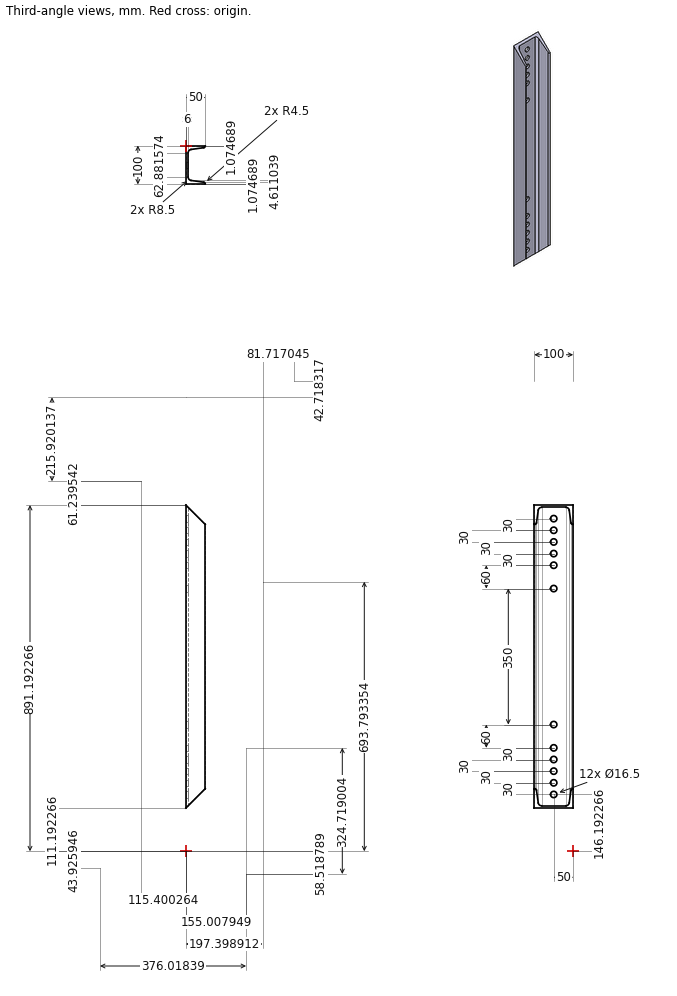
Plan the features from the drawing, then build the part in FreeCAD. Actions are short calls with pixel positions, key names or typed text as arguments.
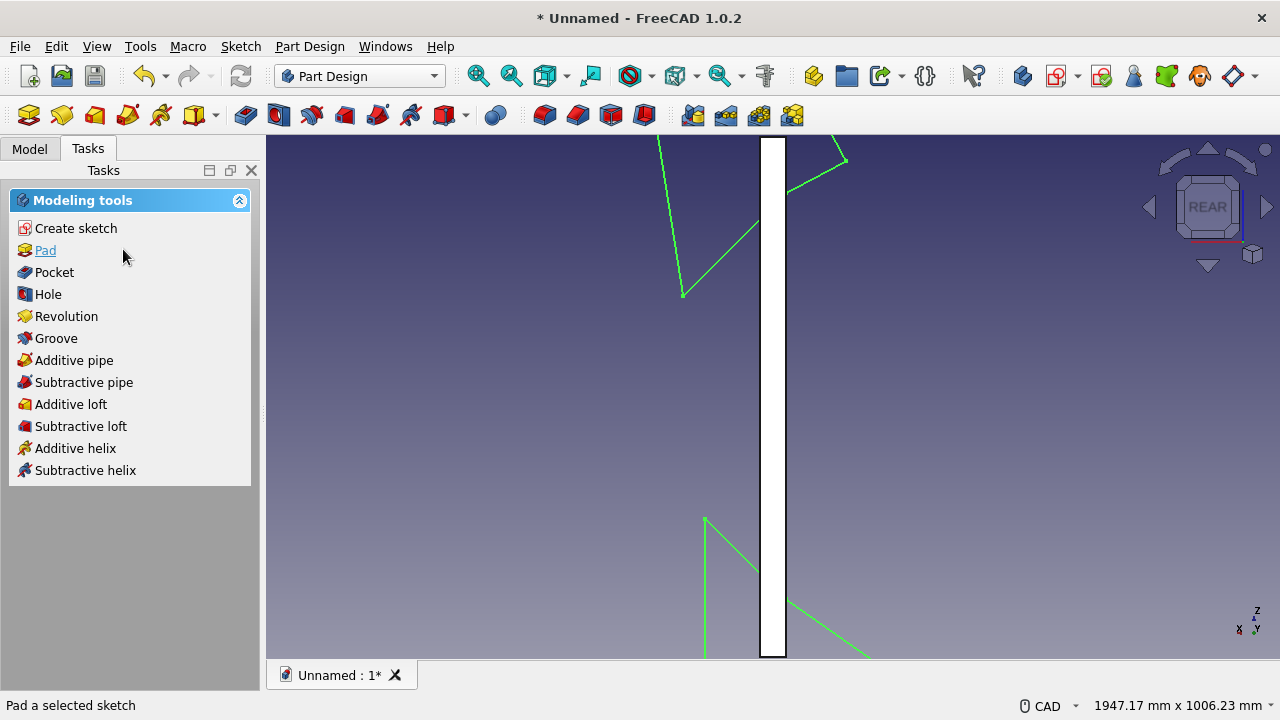
click(246, 116)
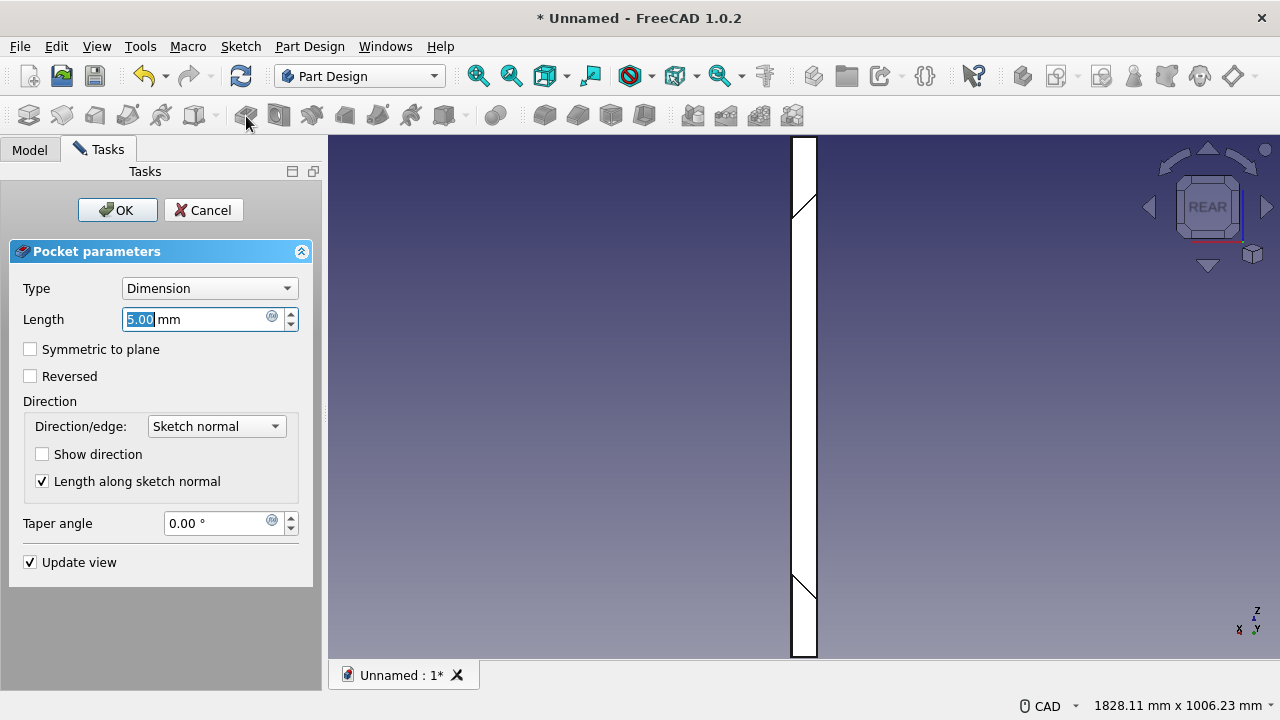
text(100)
key(Tab)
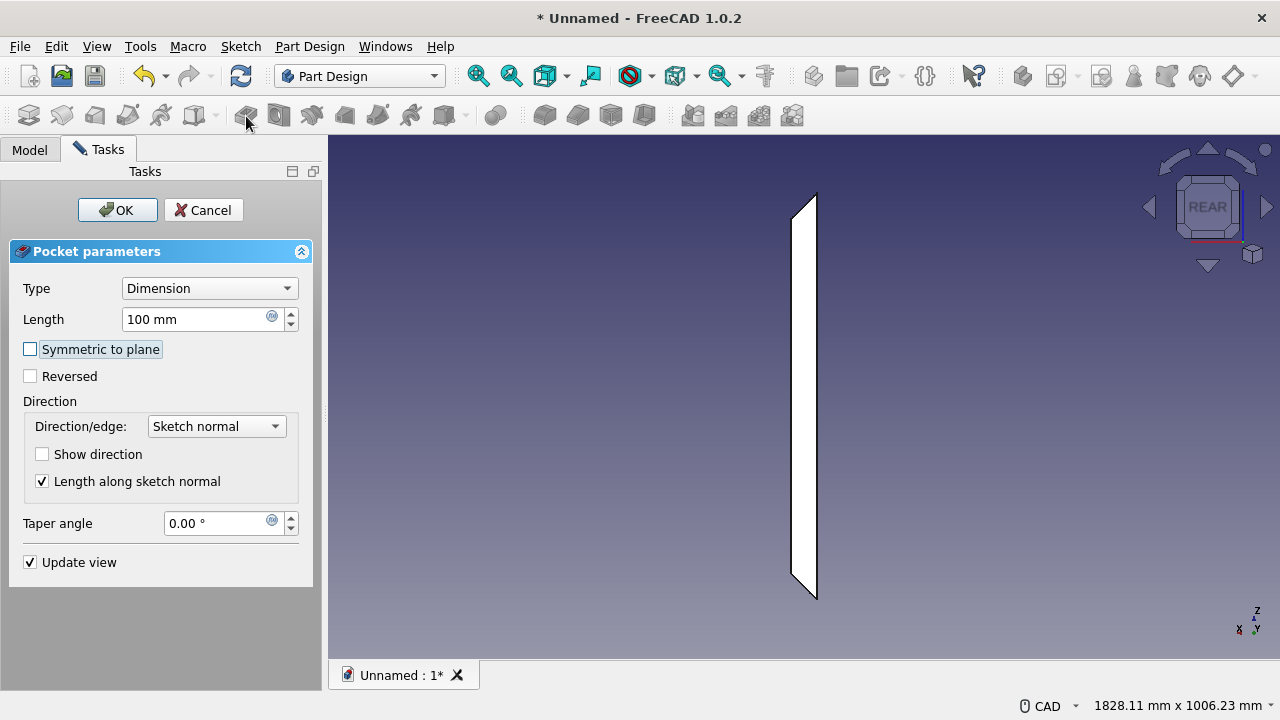
click(118, 210)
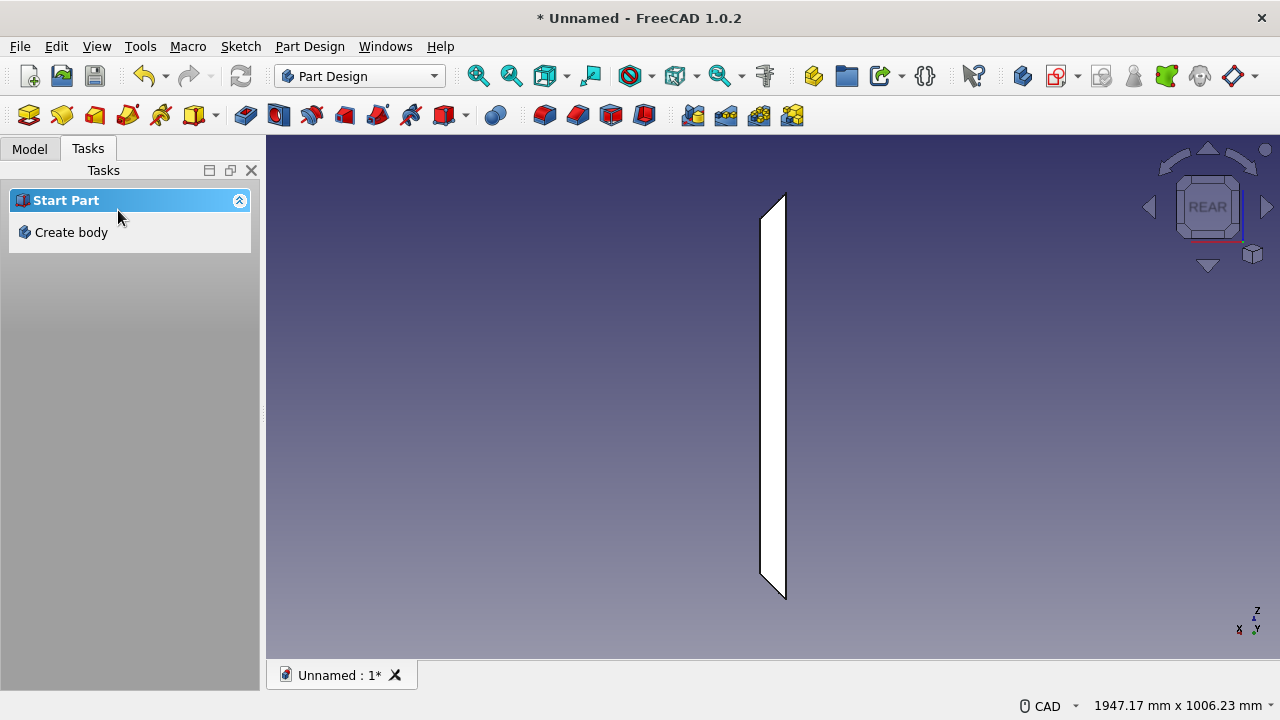
key(6)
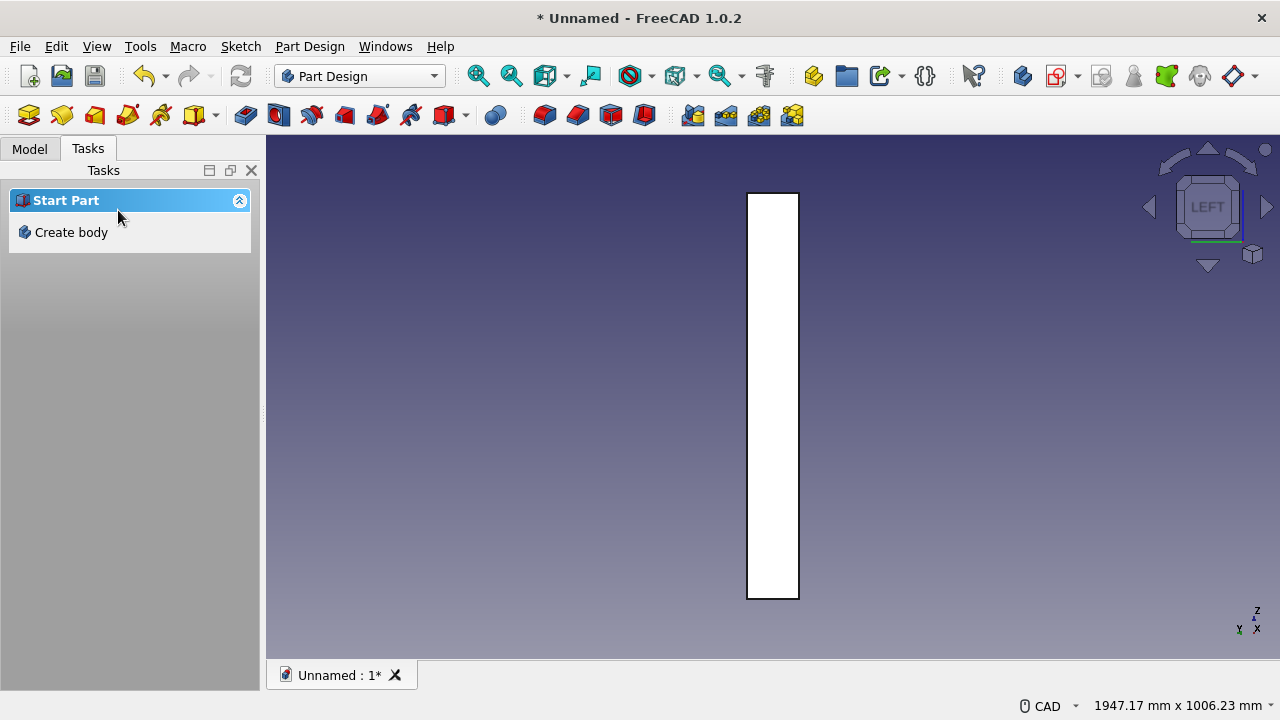
click(773, 221)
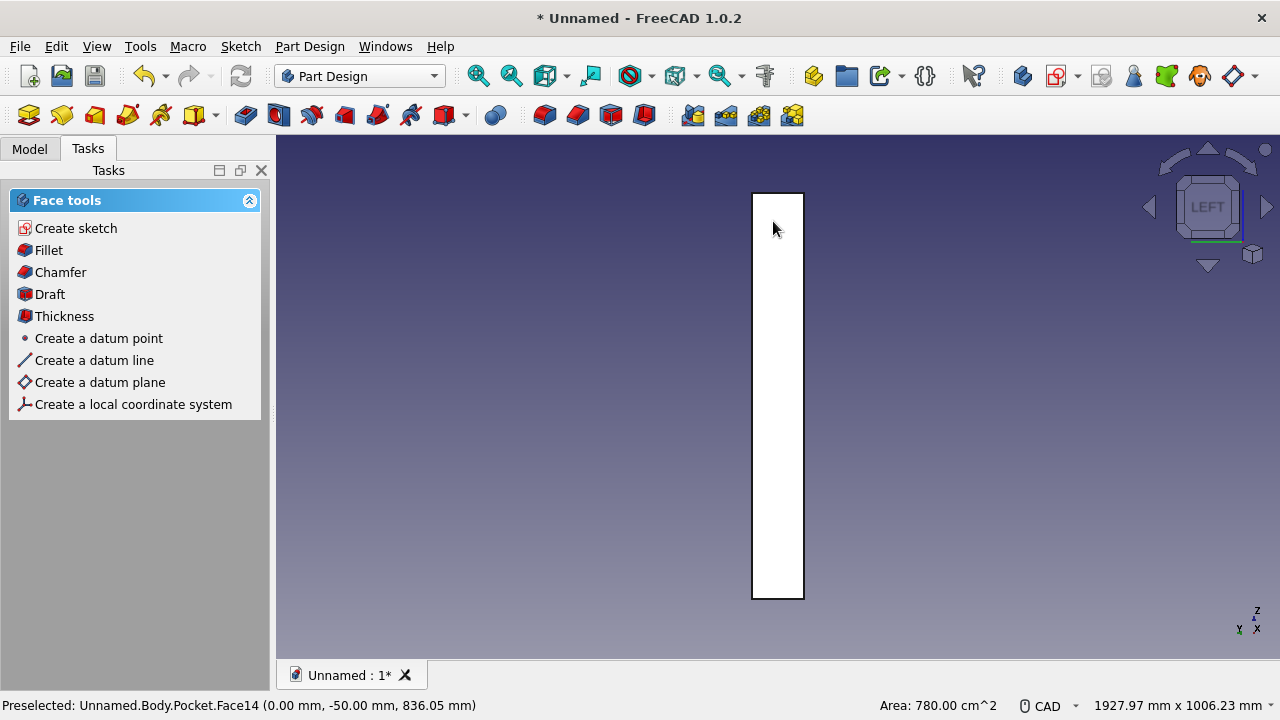
click(1056, 76)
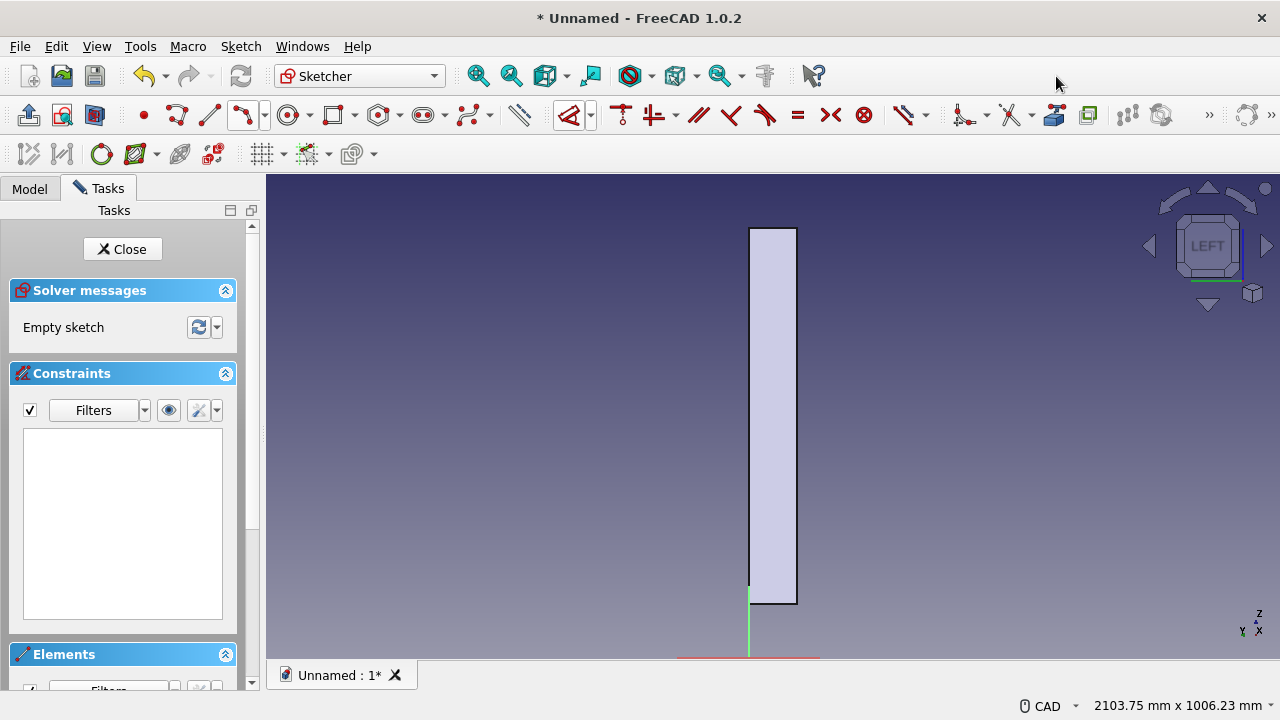
scroll(586, 350, down, 2)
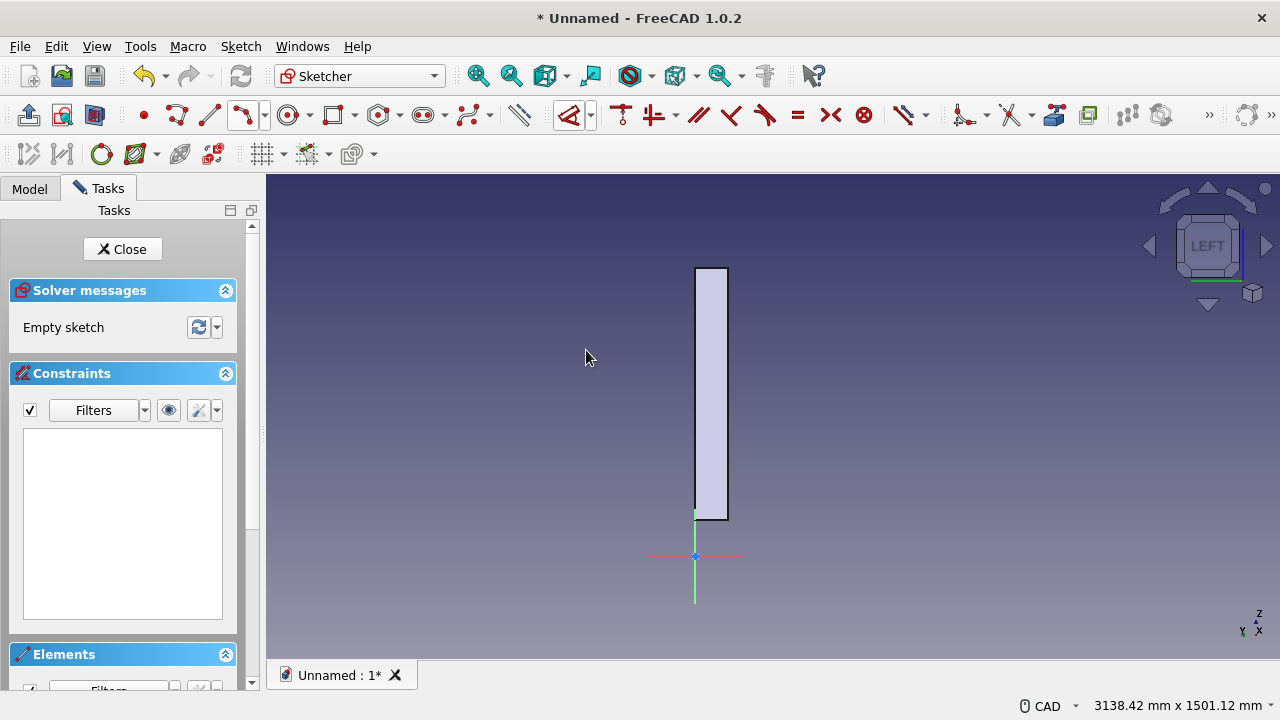
click(288, 116)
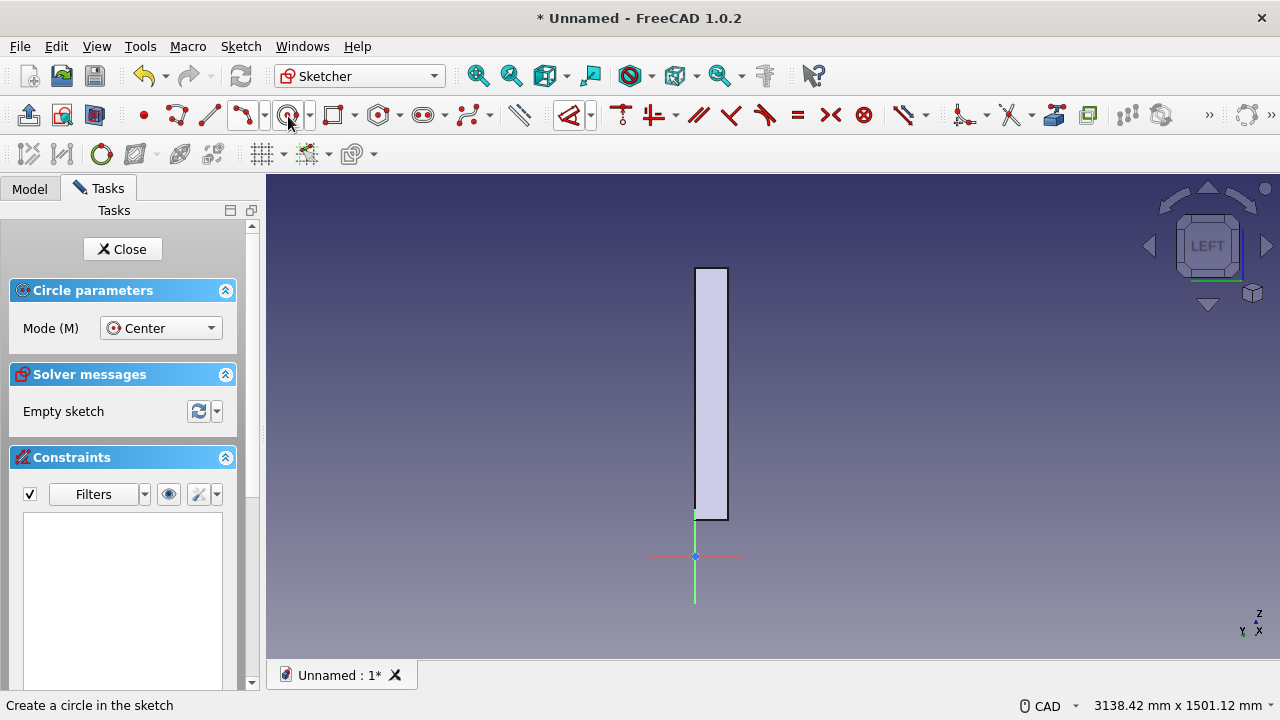
scroll(711, 509, up, 11)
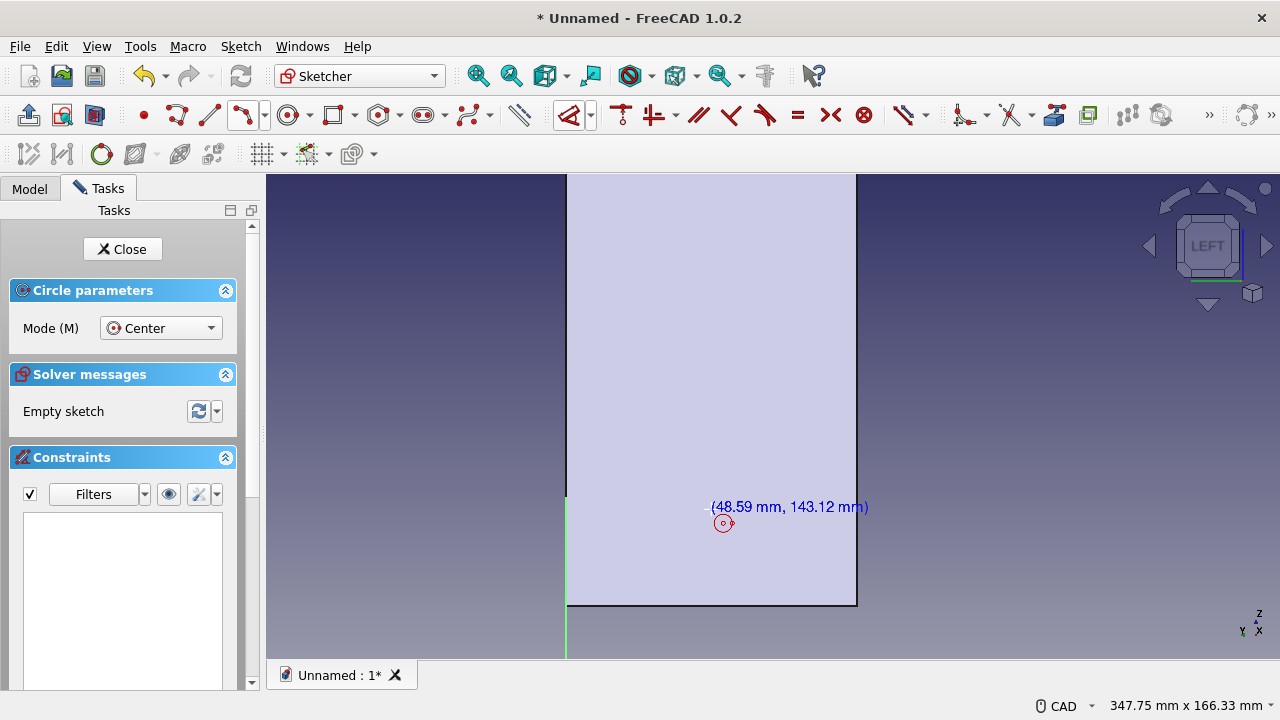
scroll(711, 510, down, 11)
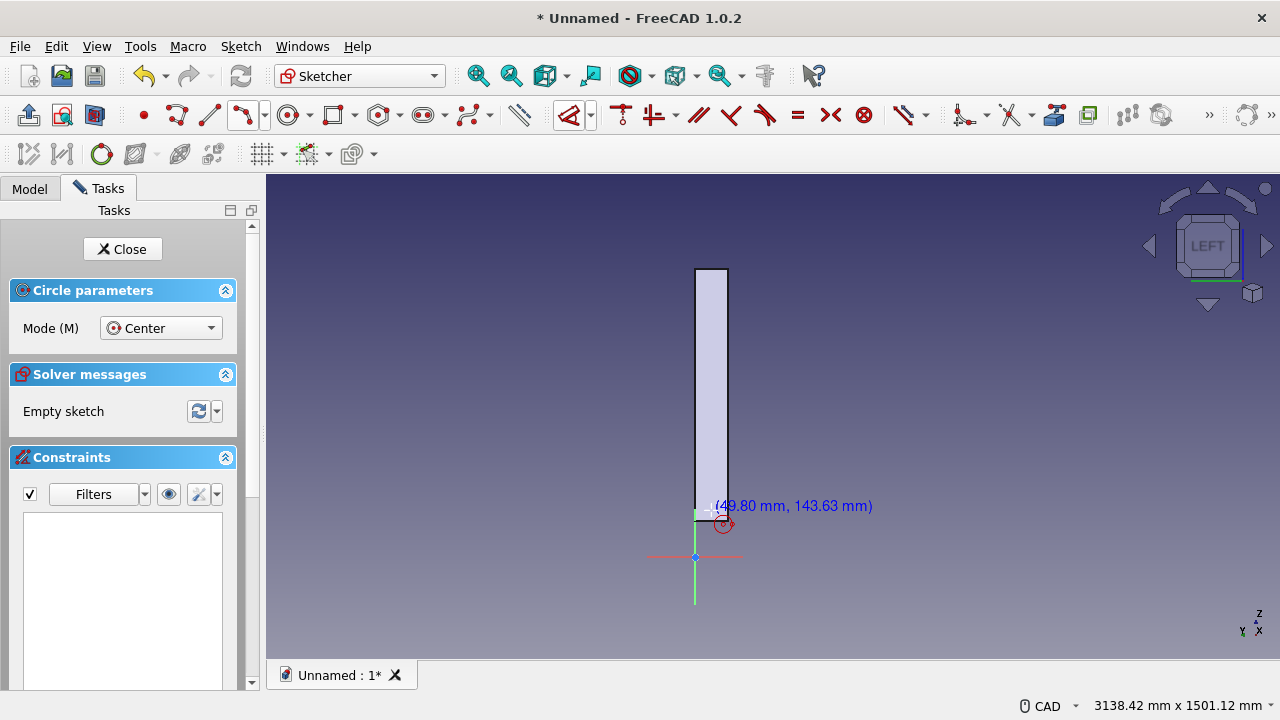
click(711, 510)
move(713, 508)